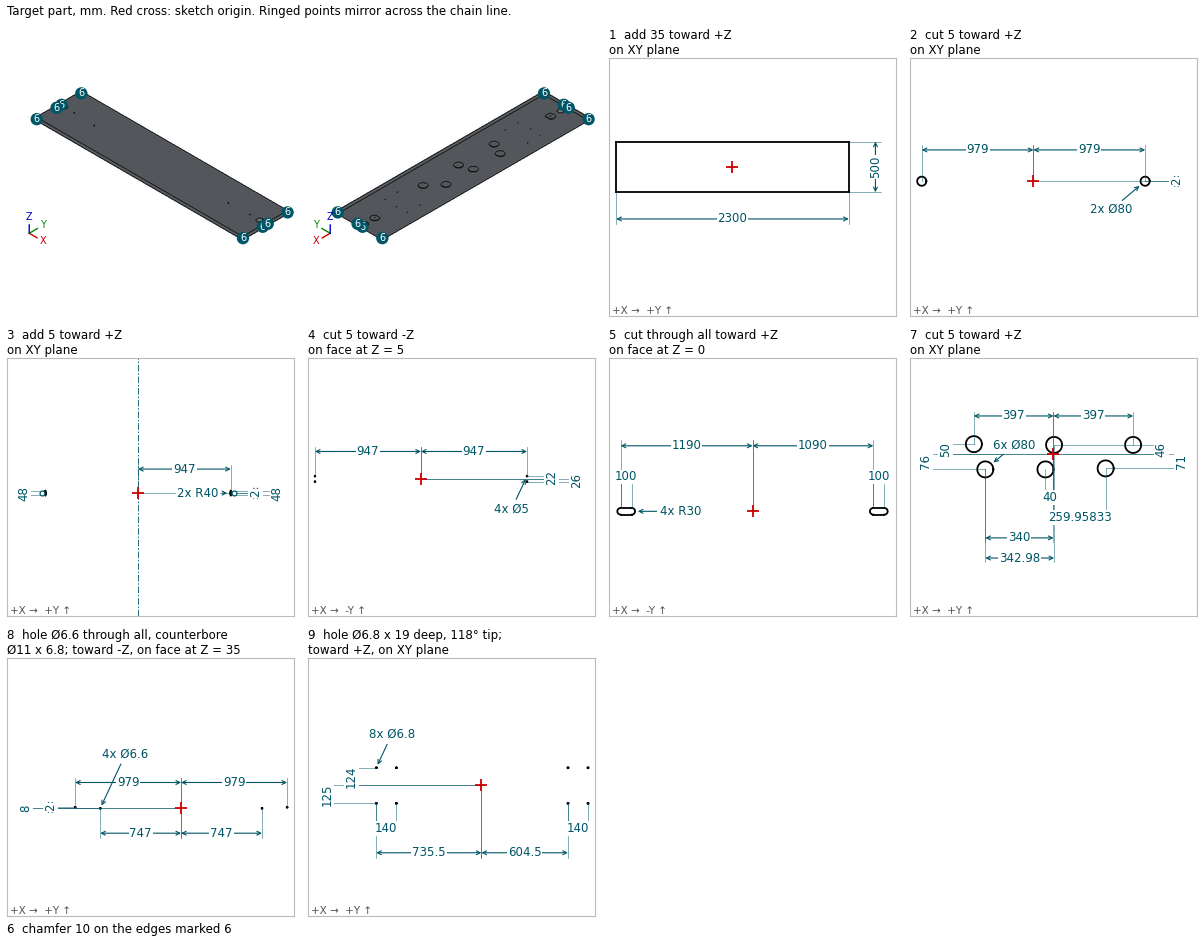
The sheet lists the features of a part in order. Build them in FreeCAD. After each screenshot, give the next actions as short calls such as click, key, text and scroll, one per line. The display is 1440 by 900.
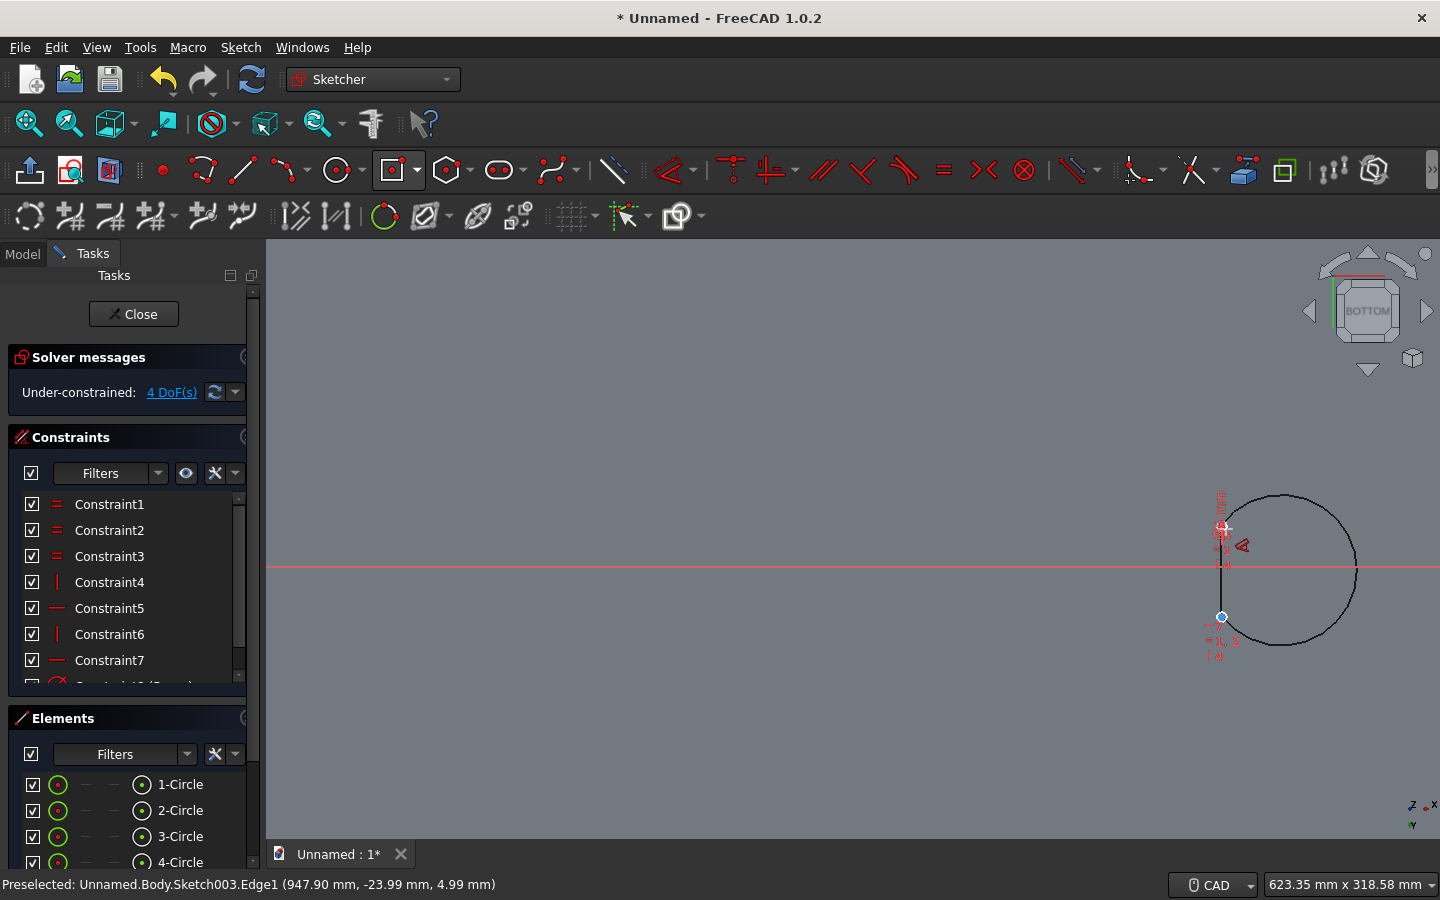
click(1222, 526)
click(1256, 546)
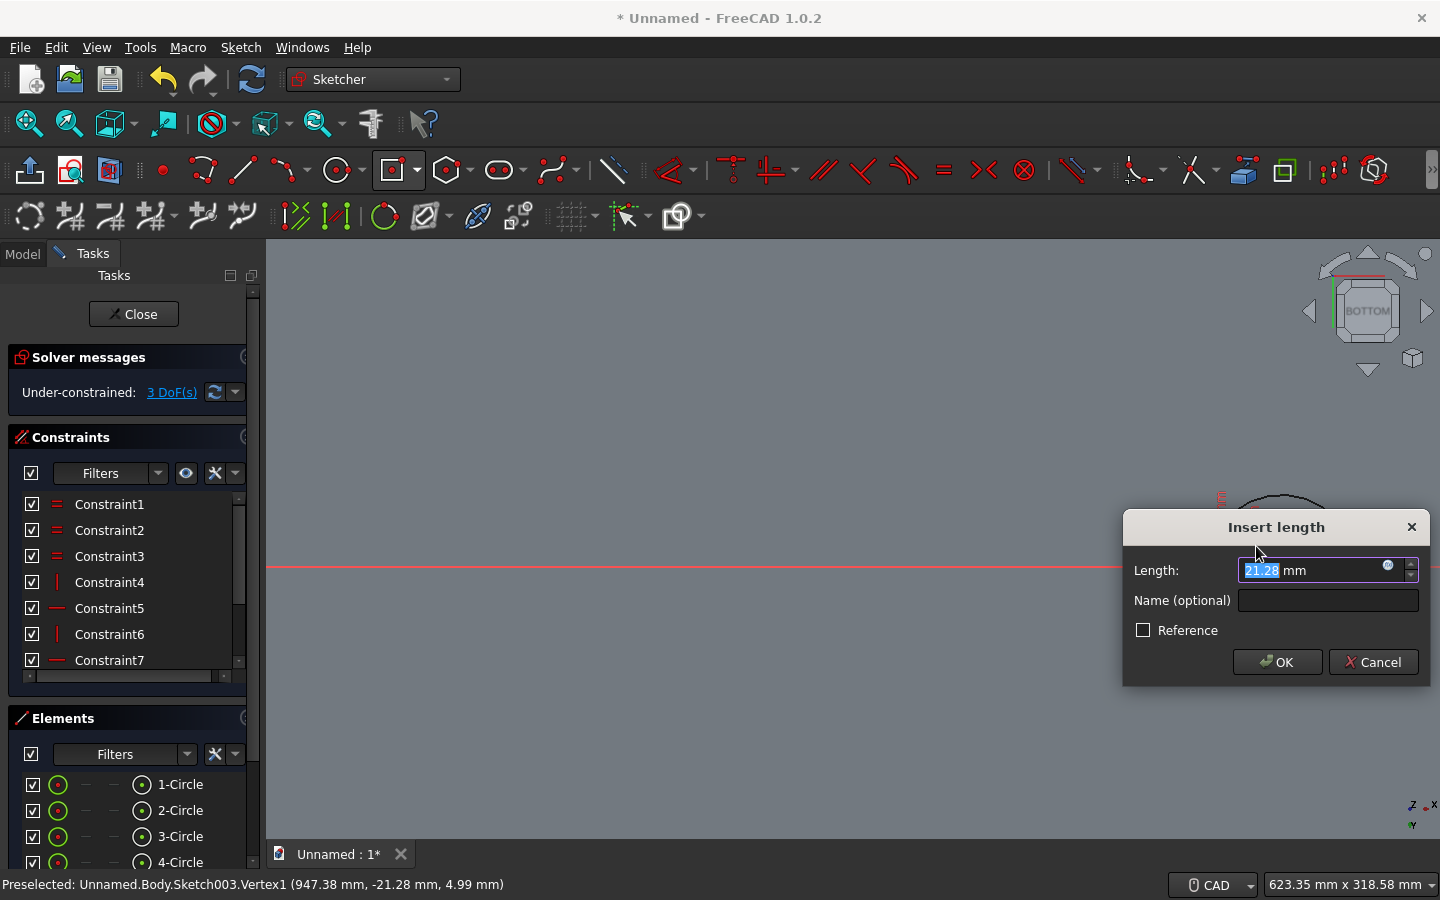
text(22)
key(Return)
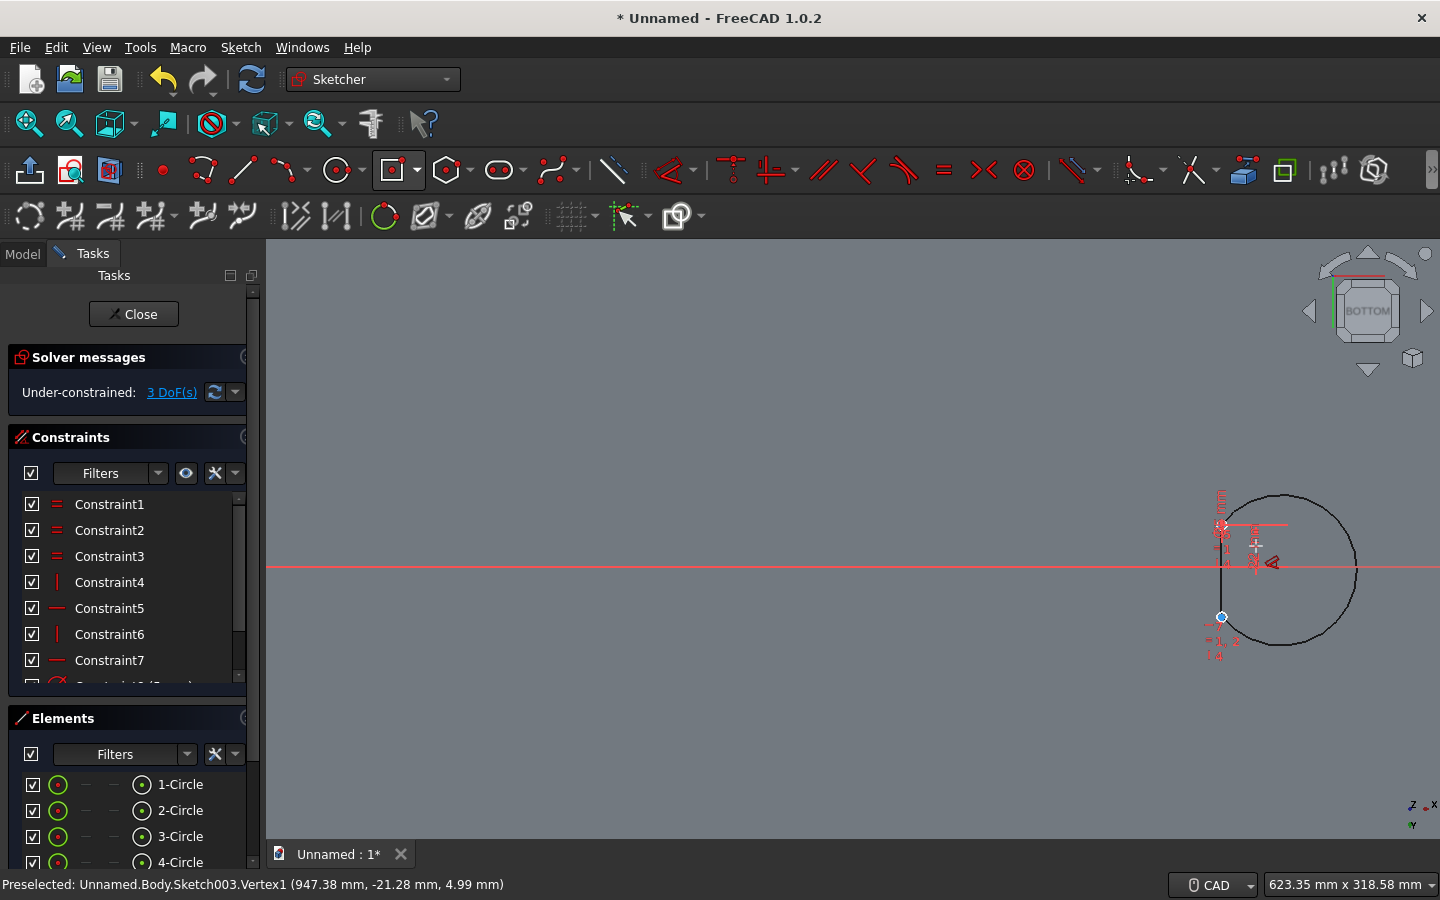
click(1222, 617)
click(1256, 592)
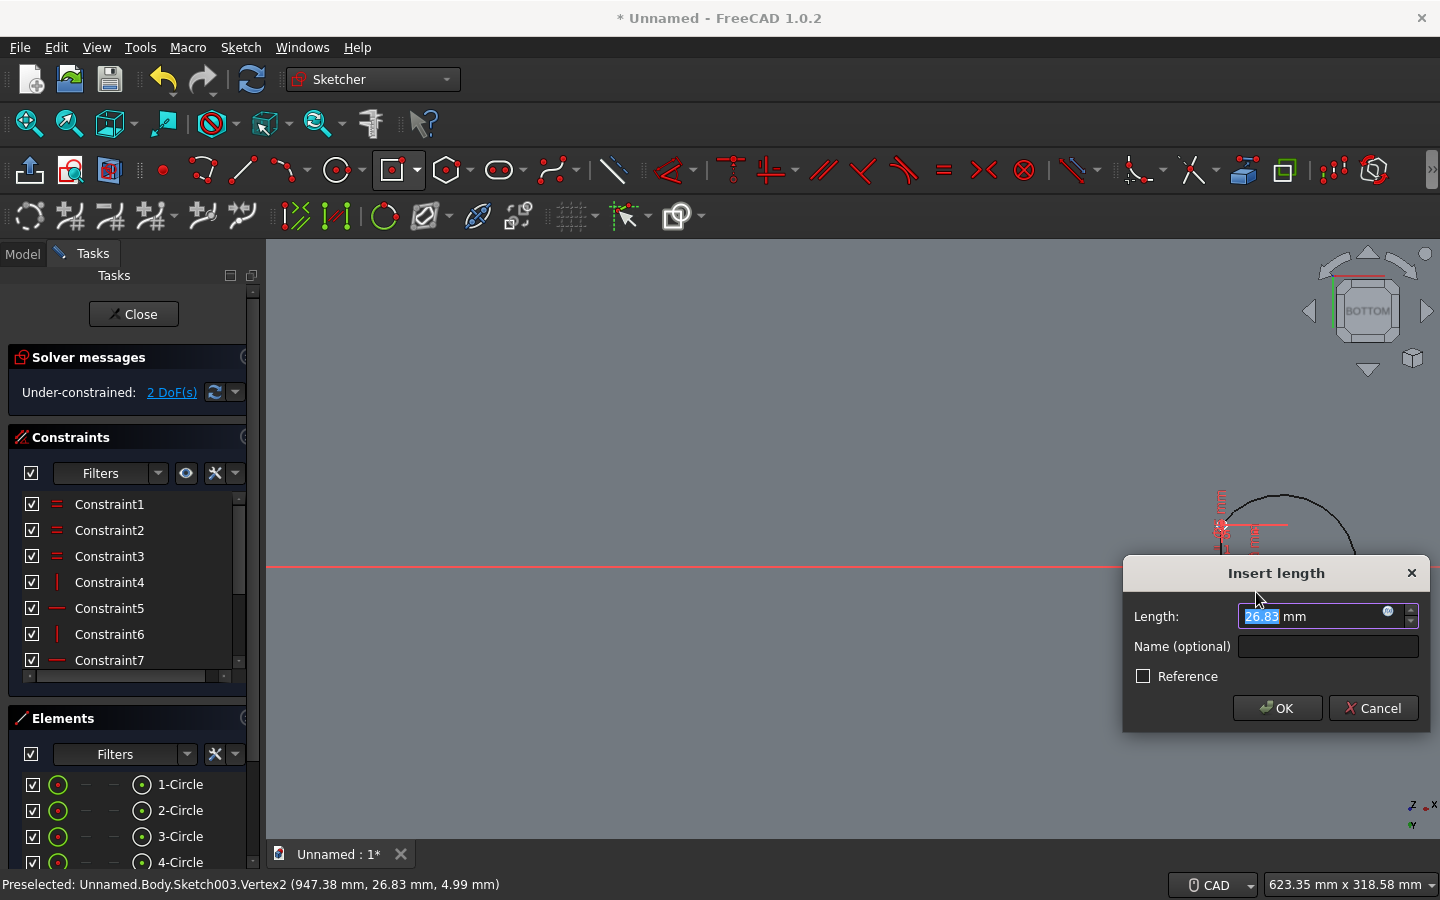
text(26)
key(Return)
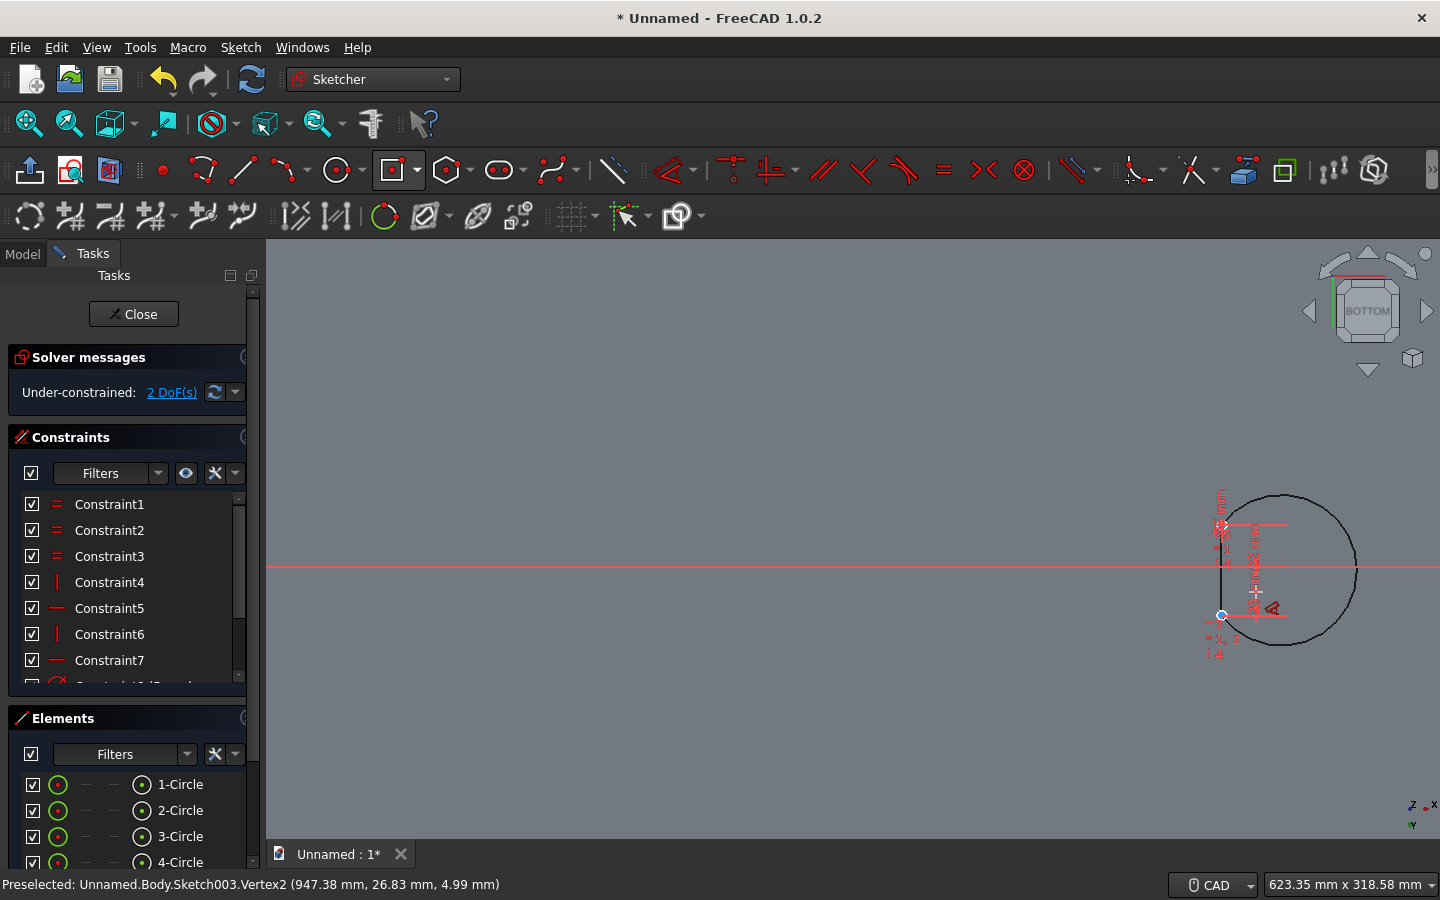
scroll(1125, 531, down, 8)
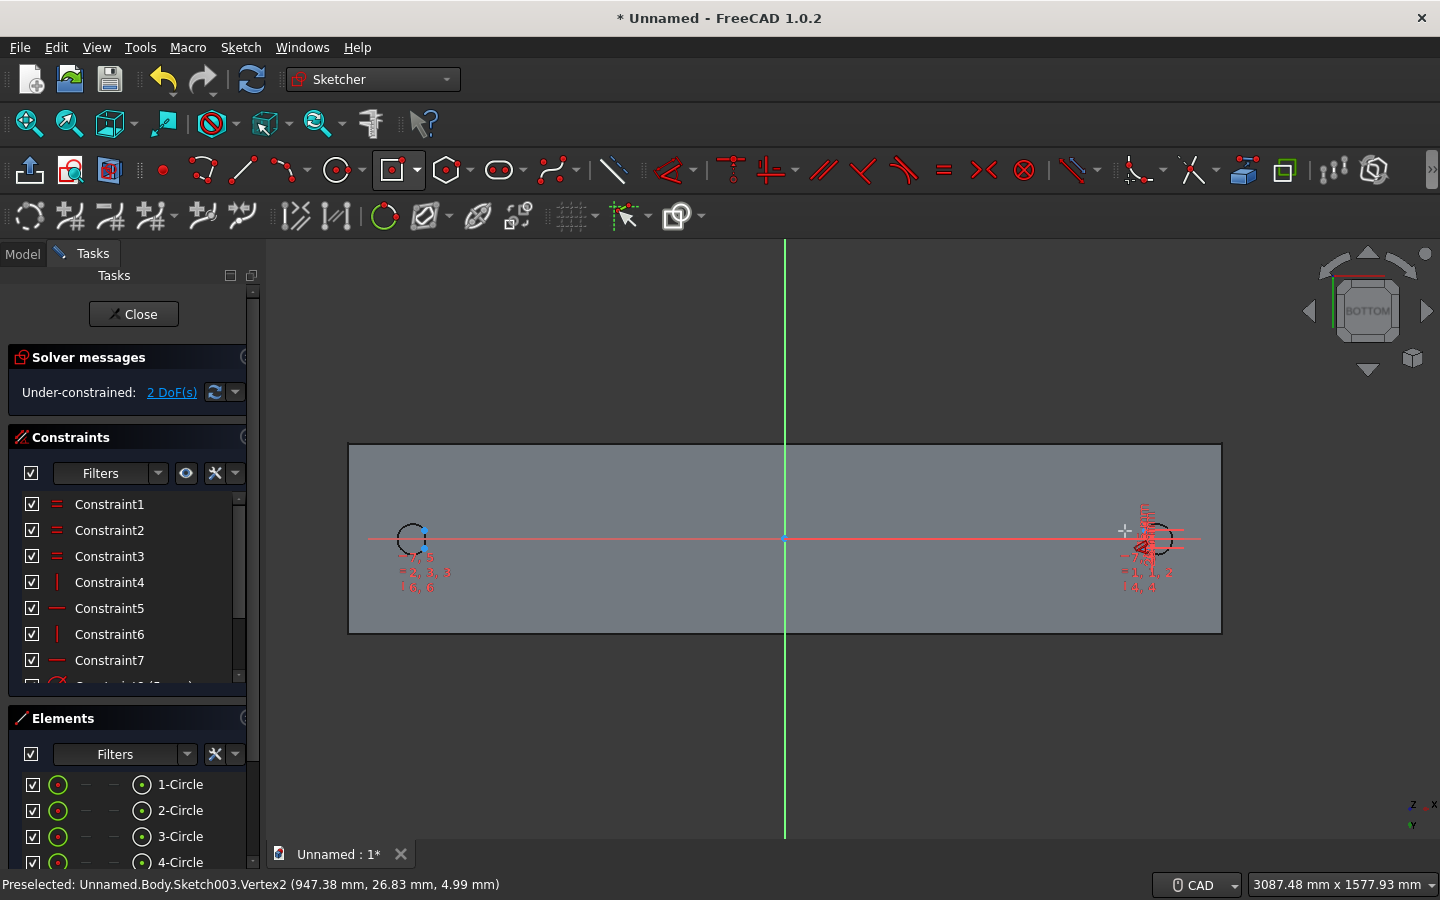
click(1145, 530)
click(965, 496)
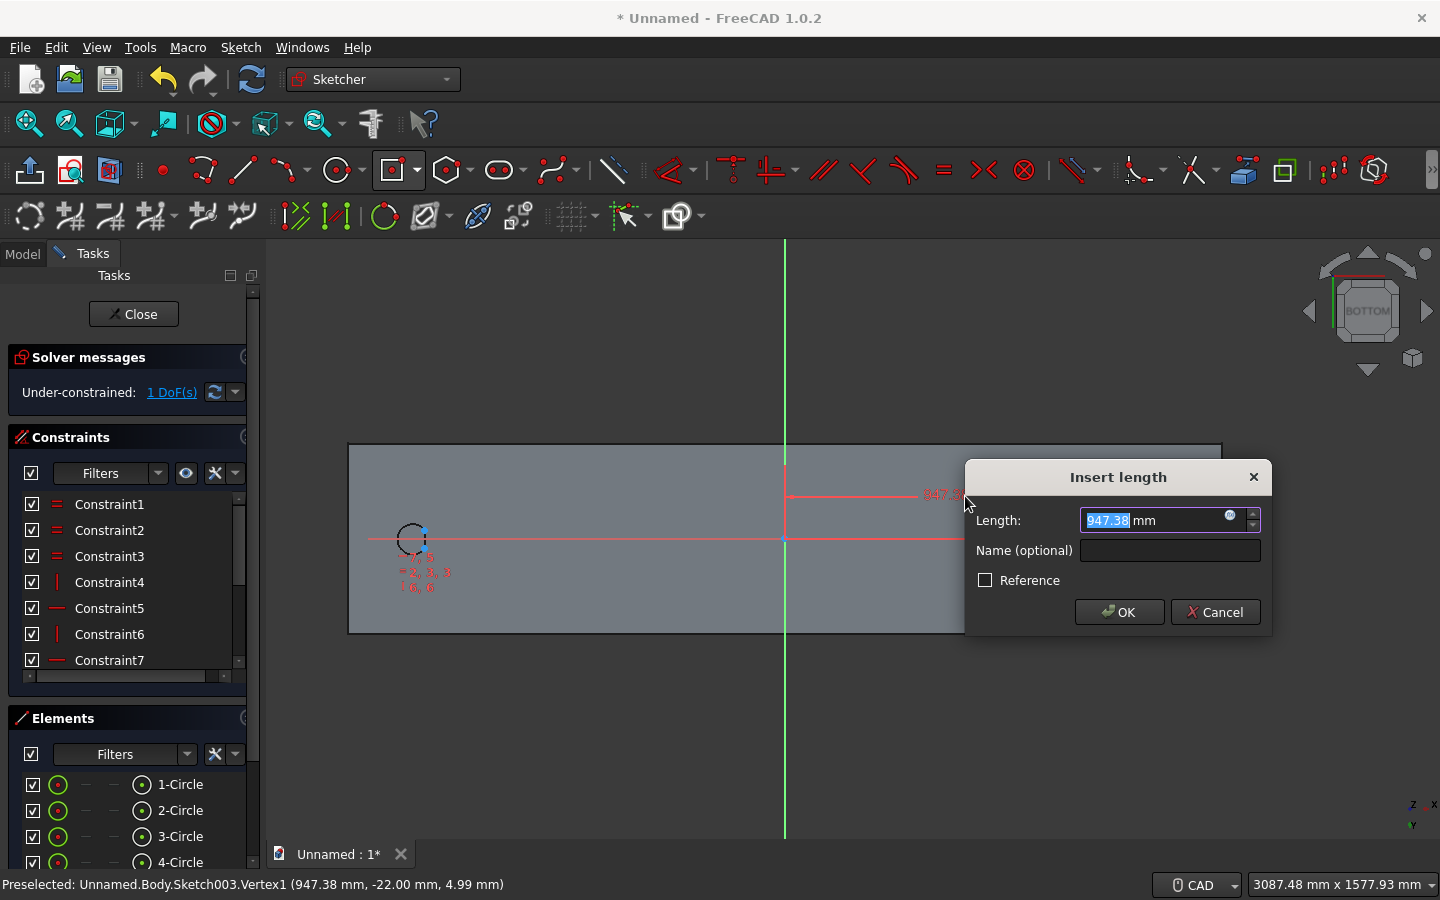
text(947)
key(Return)